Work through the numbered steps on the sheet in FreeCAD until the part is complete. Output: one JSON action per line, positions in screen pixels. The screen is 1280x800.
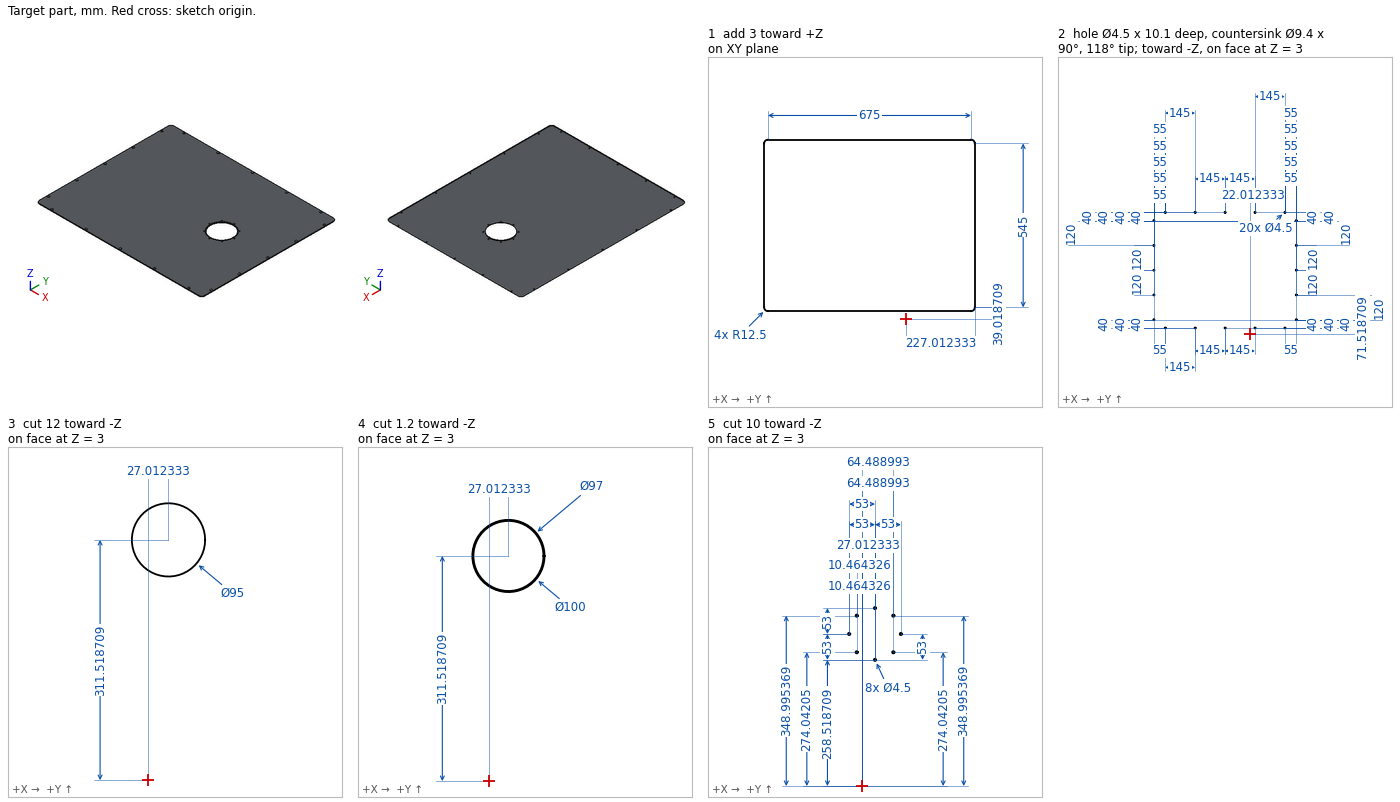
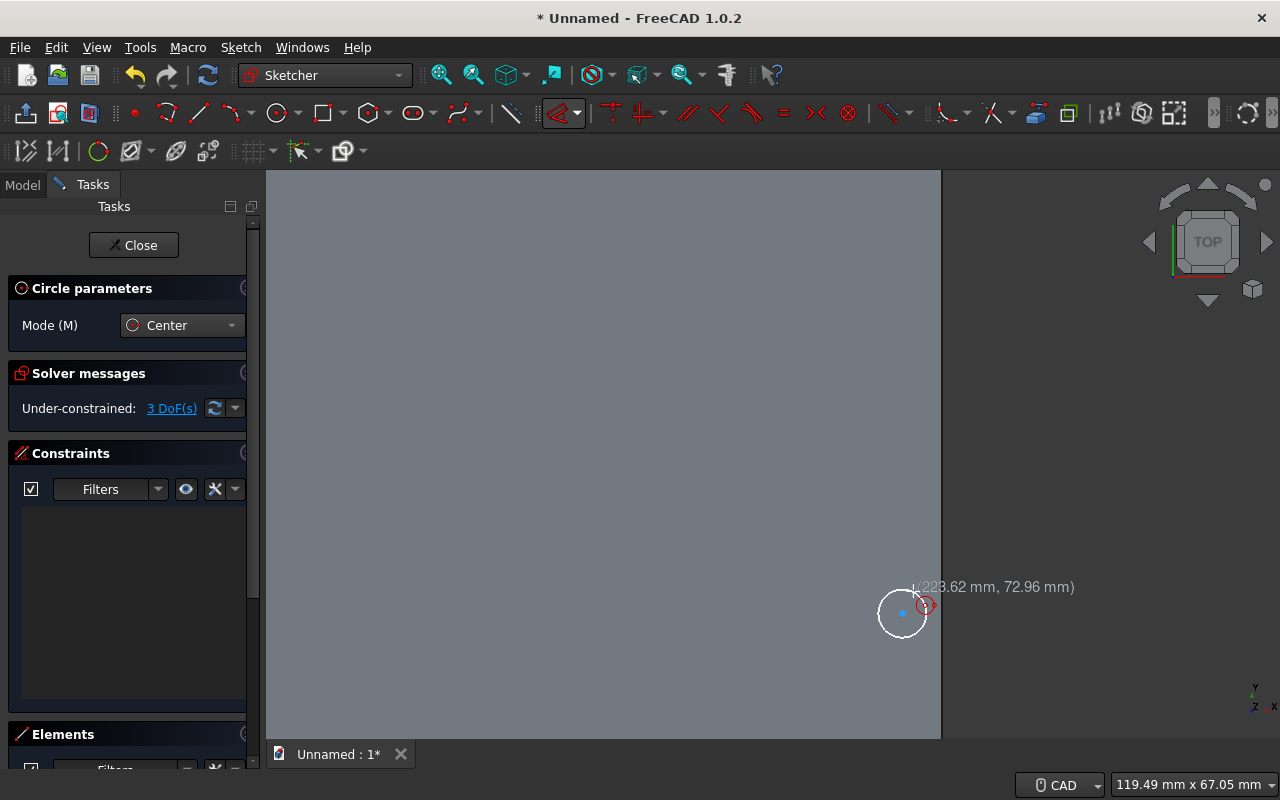
{"action": "scroll", "coordinate": [924, 596], "scroll_direction": "down", "scroll_amount": 13}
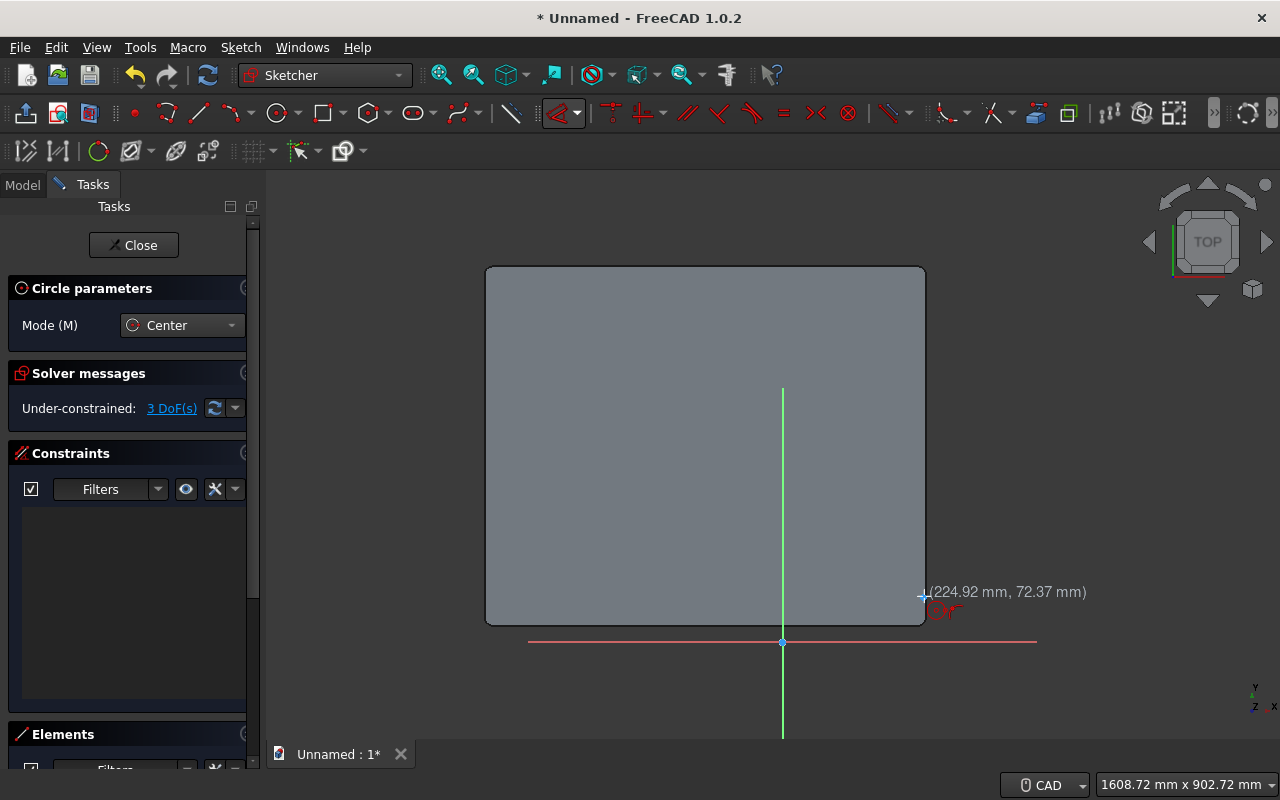
{"action": "scroll", "coordinate": [923, 522], "scroll_direction": "up", "scroll_amount": 14}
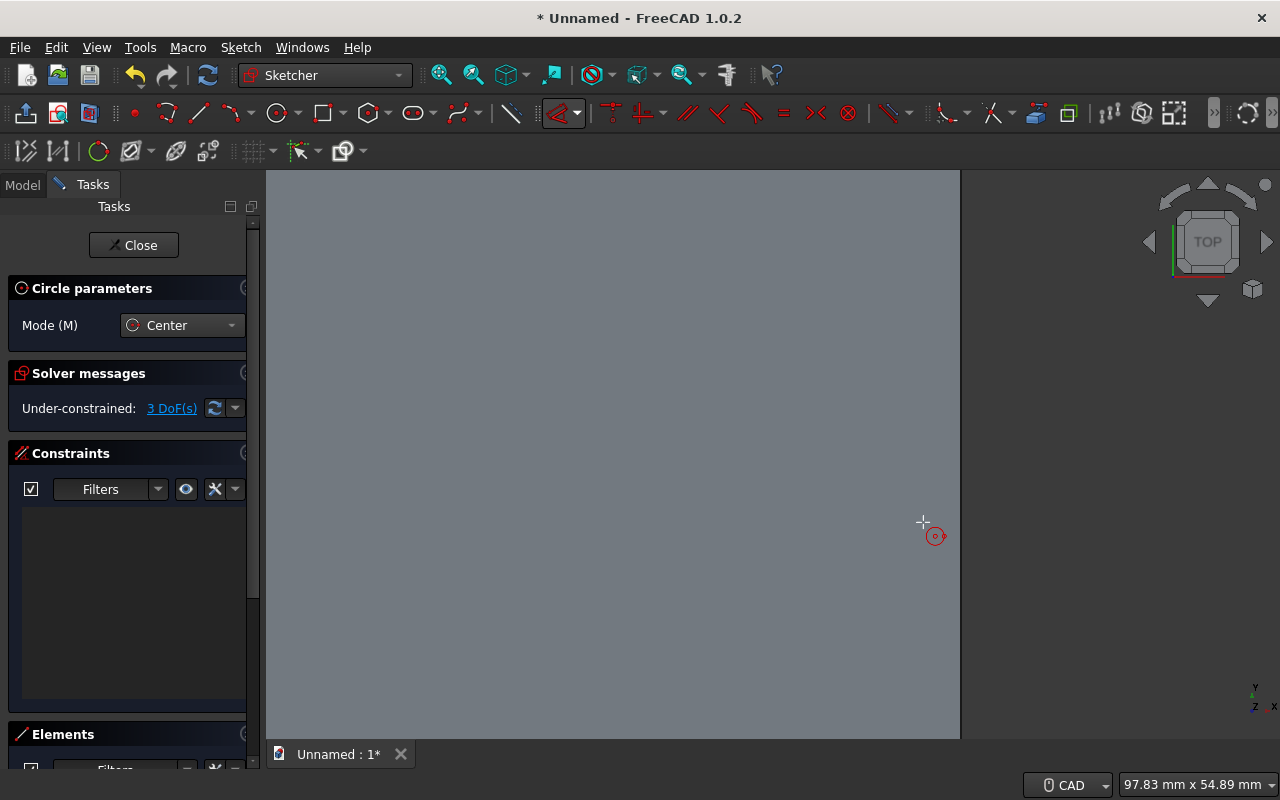
{"action": "scroll", "coordinate": [923, 522], "scroll_direction": "down", "scroll_amount": 14}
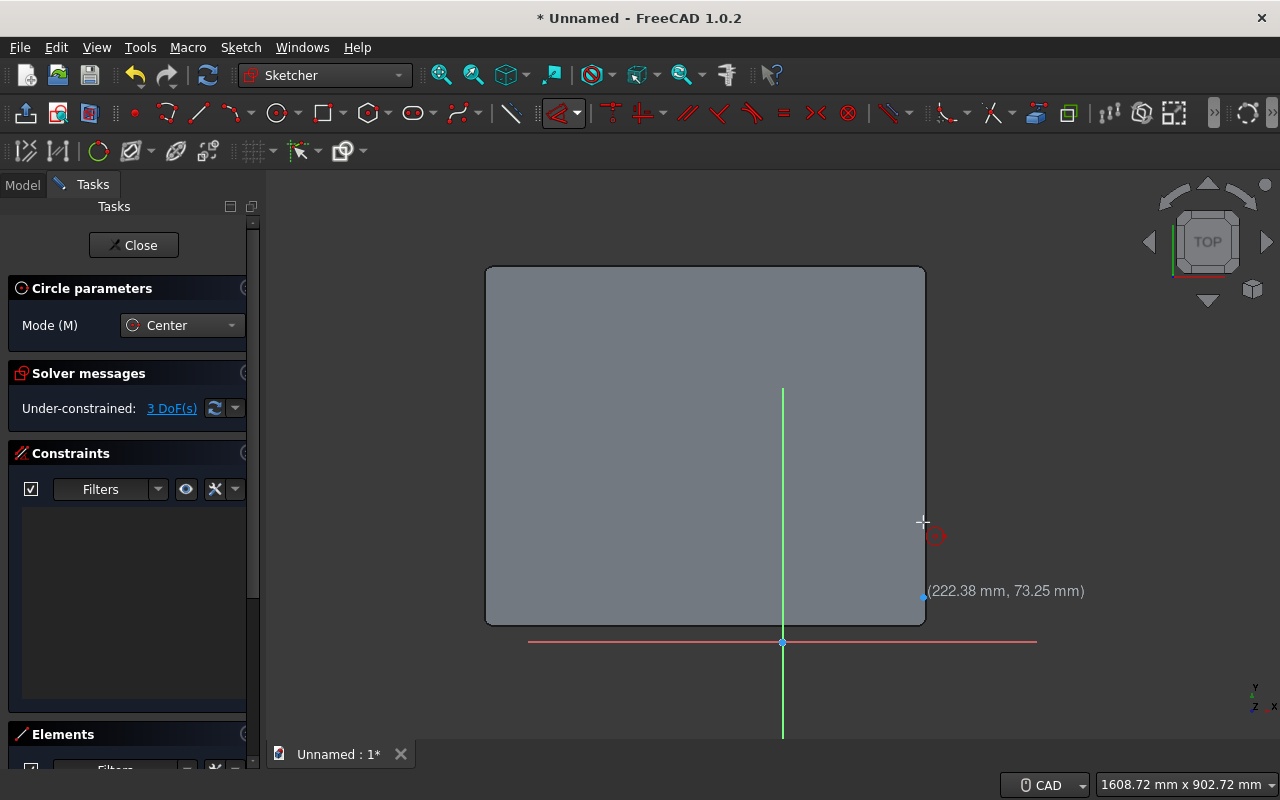
{"action": "left_click", "coordinate": [923, 522]}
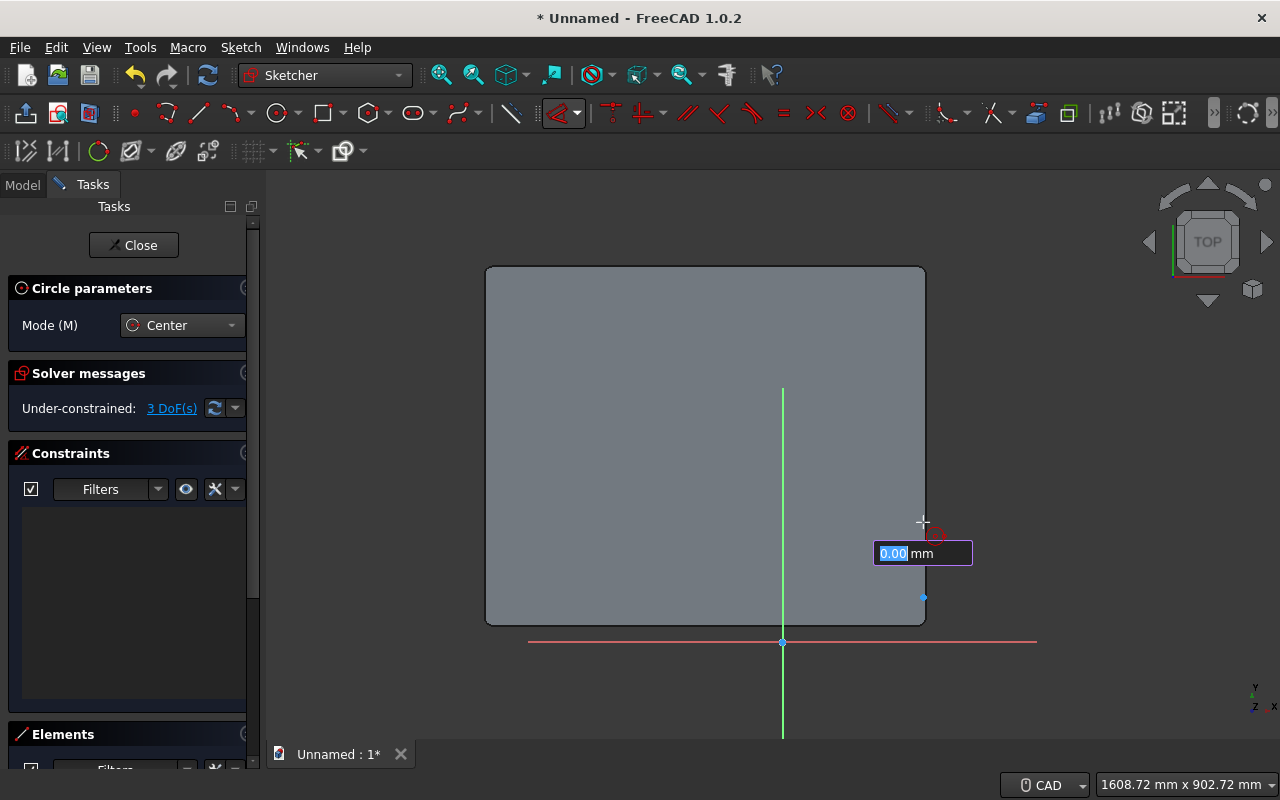
{"action": "scroll", "coordinate": [924, 521], "scroll_direction": "up", "scroll_amount": 13}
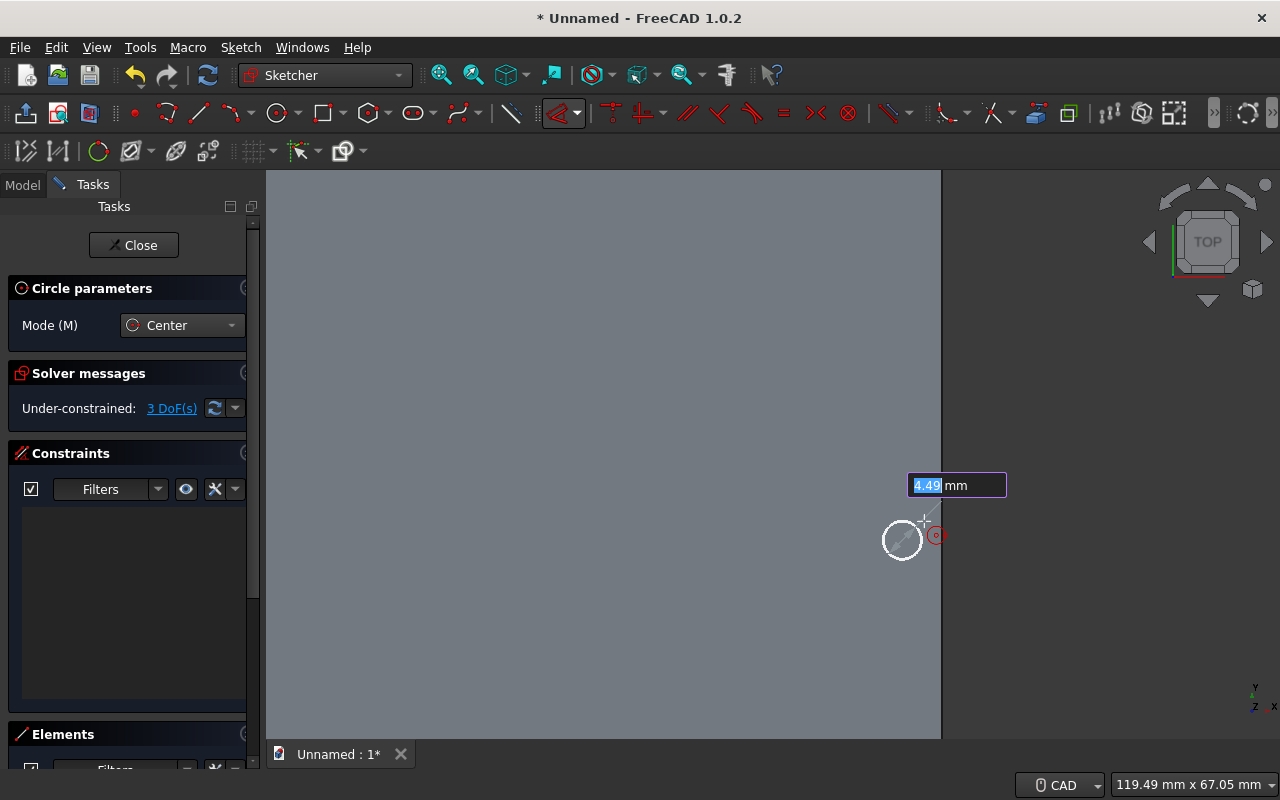
{"action": "left_click", "coordinate": [913, 509]}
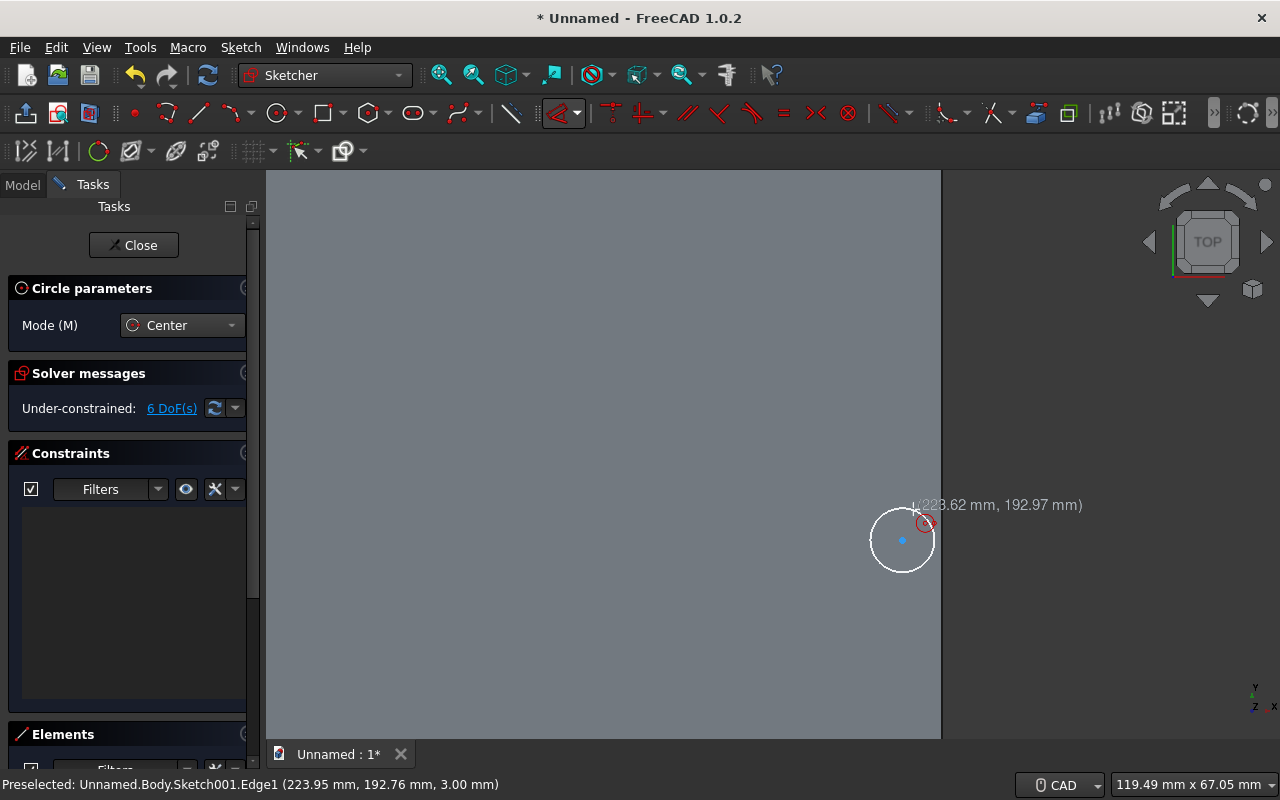
{"action": "scroll", "coordinate": [924, 521], "scroll_direction": "down", "scroll_amount": 13}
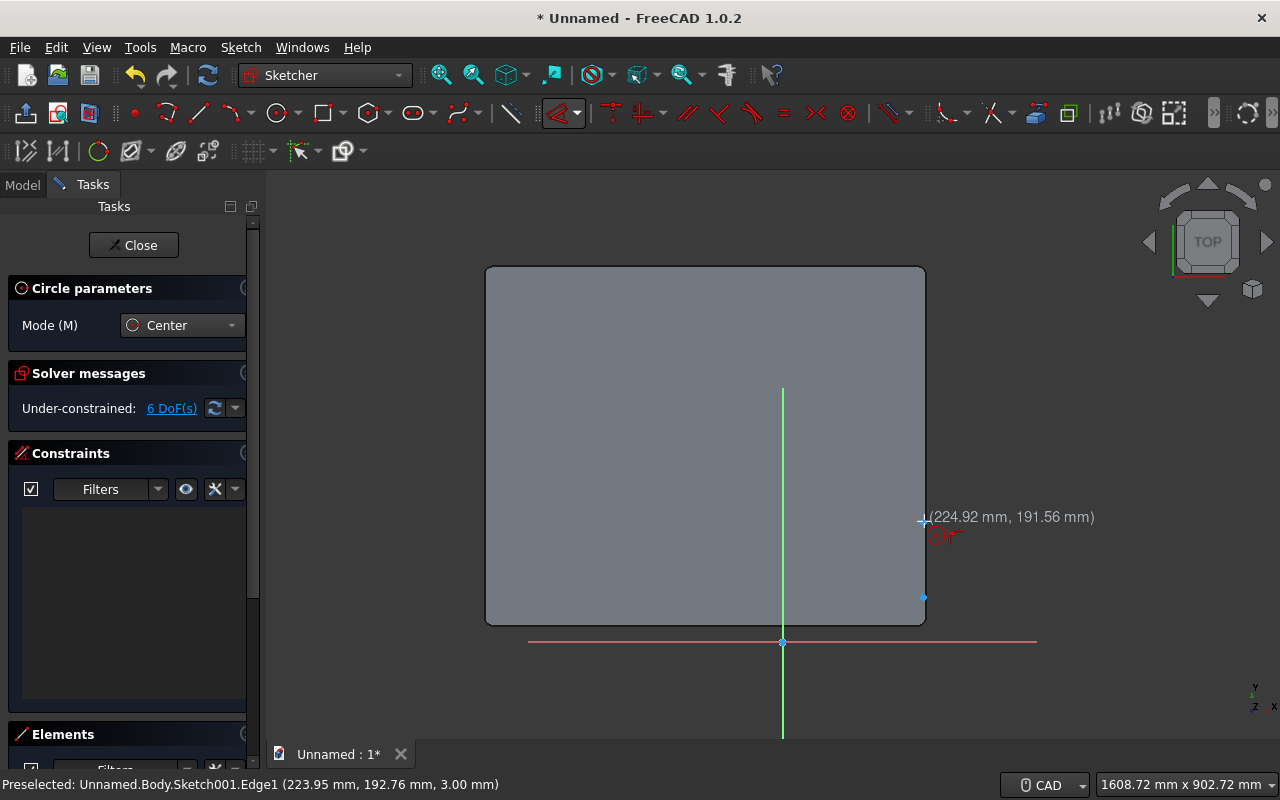
{"action": "scroll", "coordinate": [923, 446], "scroll_direction": "up", "scroll_amount": 14}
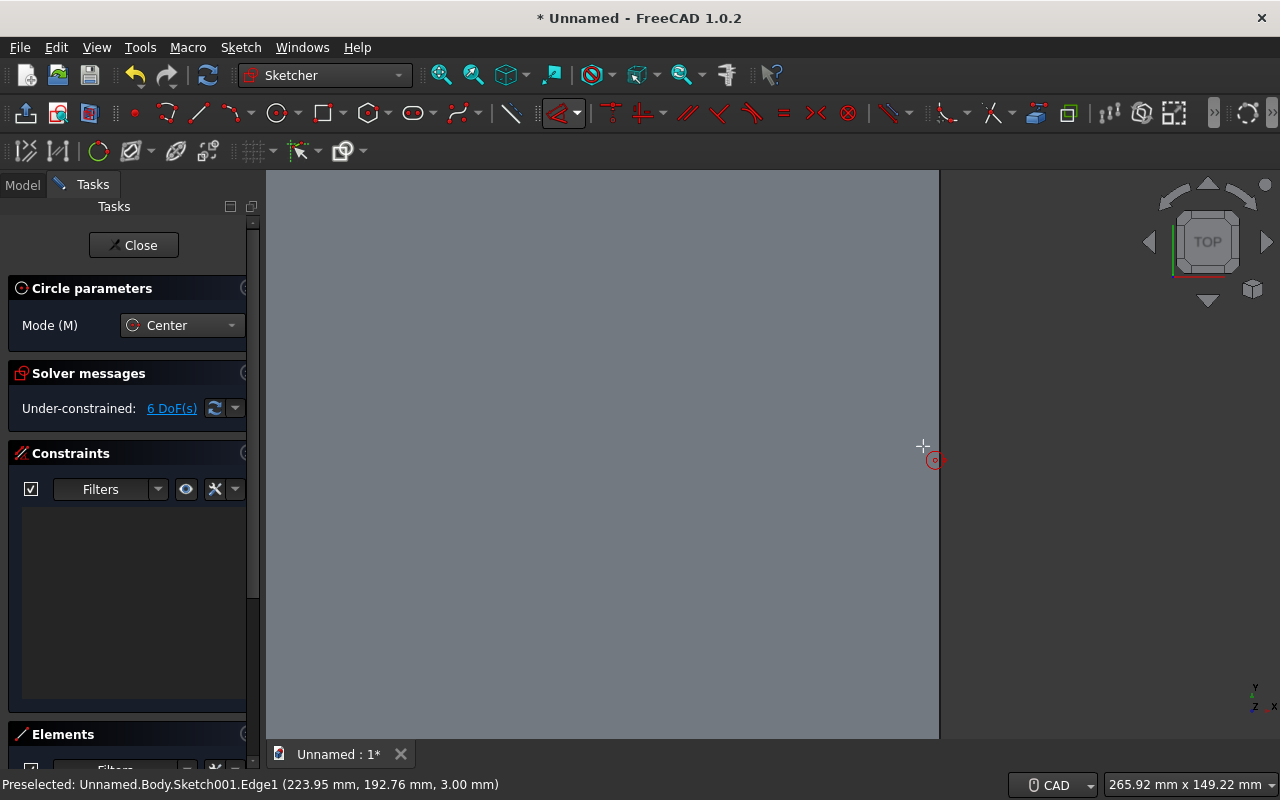
{"action": "scroll", "coordinate": [923, 446], "scroll_direction": "down", "scroll_amount": 14}